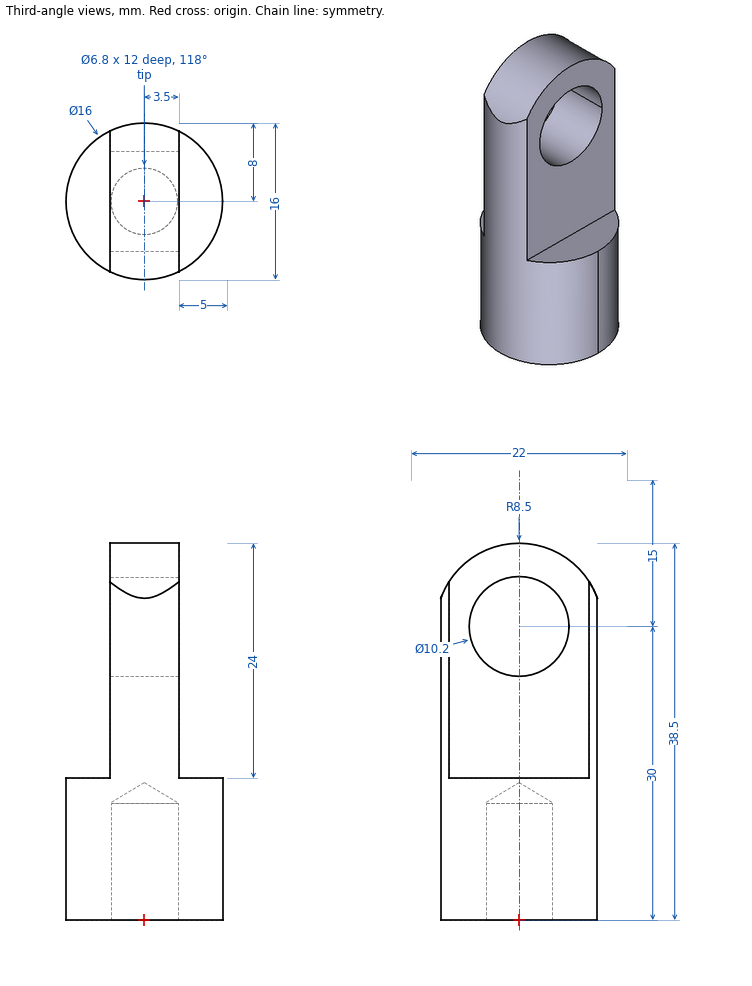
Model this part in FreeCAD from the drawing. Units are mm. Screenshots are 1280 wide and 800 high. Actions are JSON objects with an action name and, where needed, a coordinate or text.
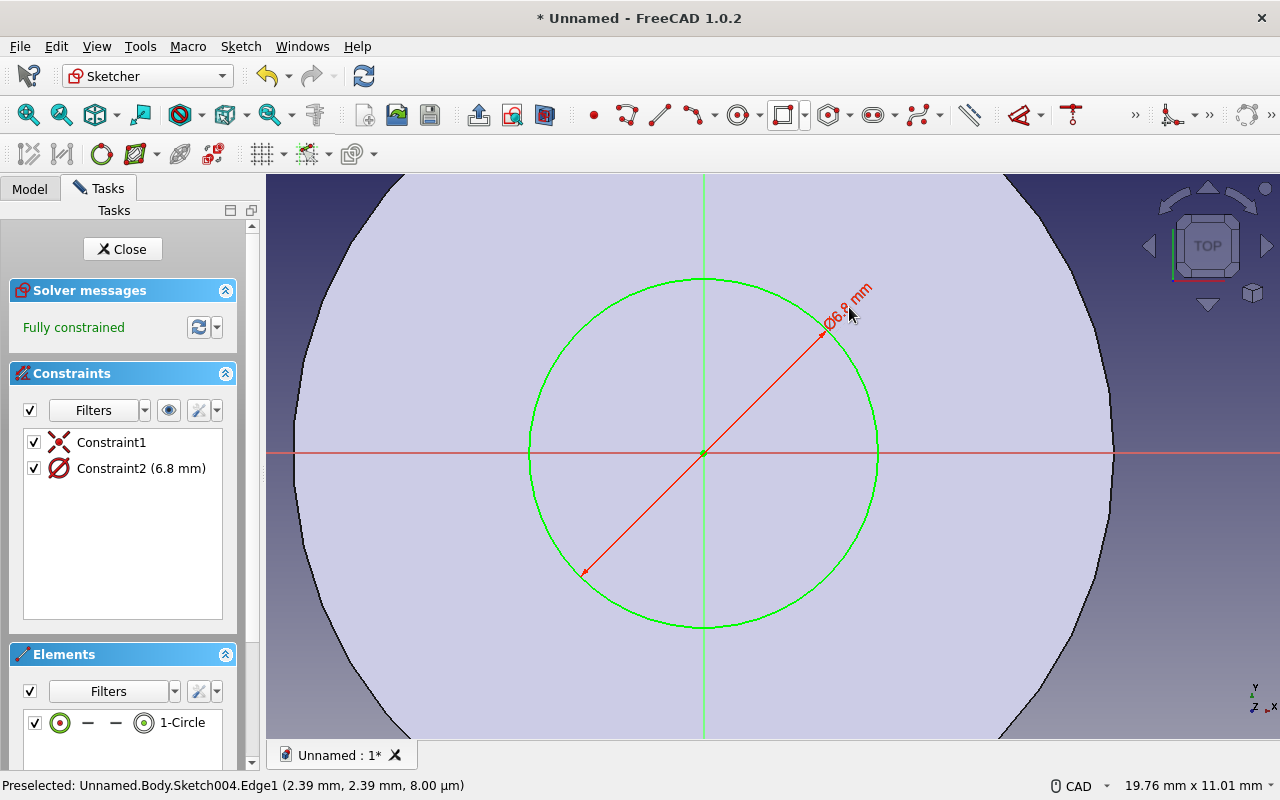
{"action": "left_click", "coordinate": [123, 249]}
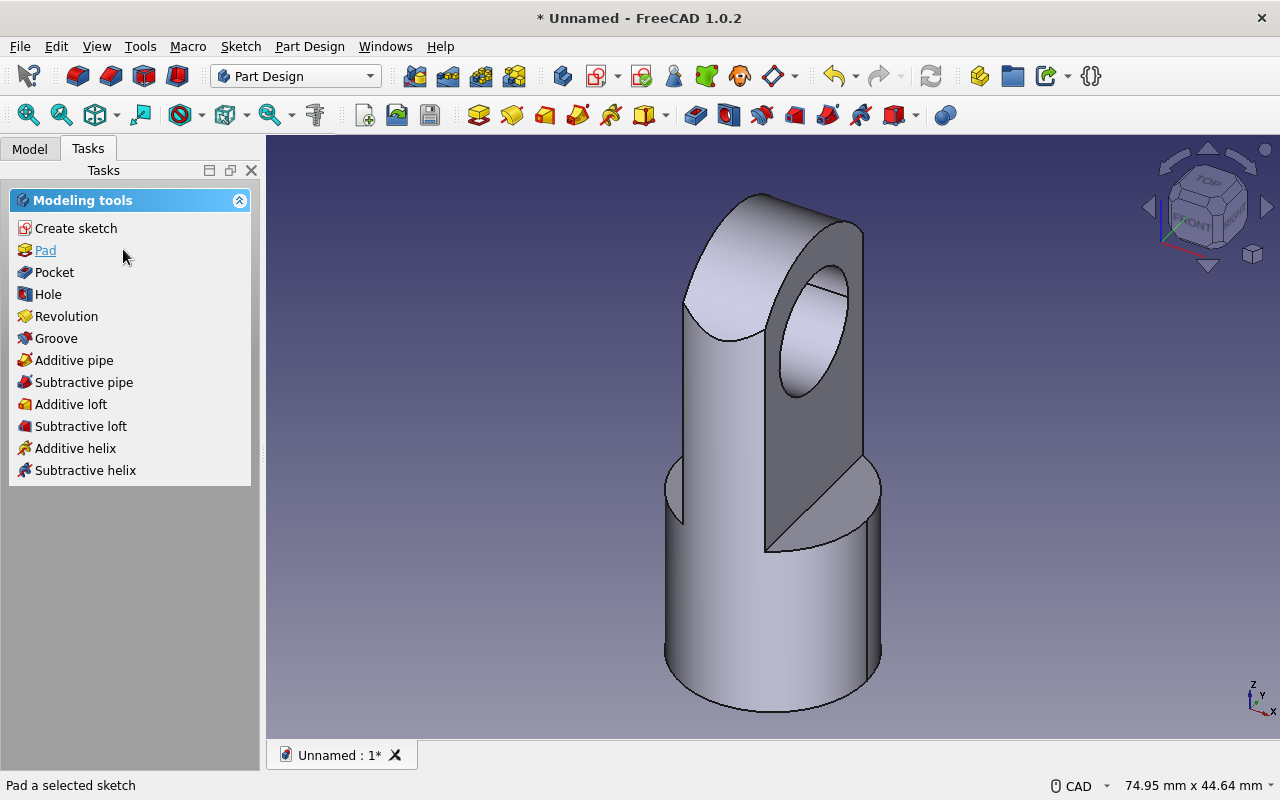
{"action": "left_click", "coordinate": [729, 116]}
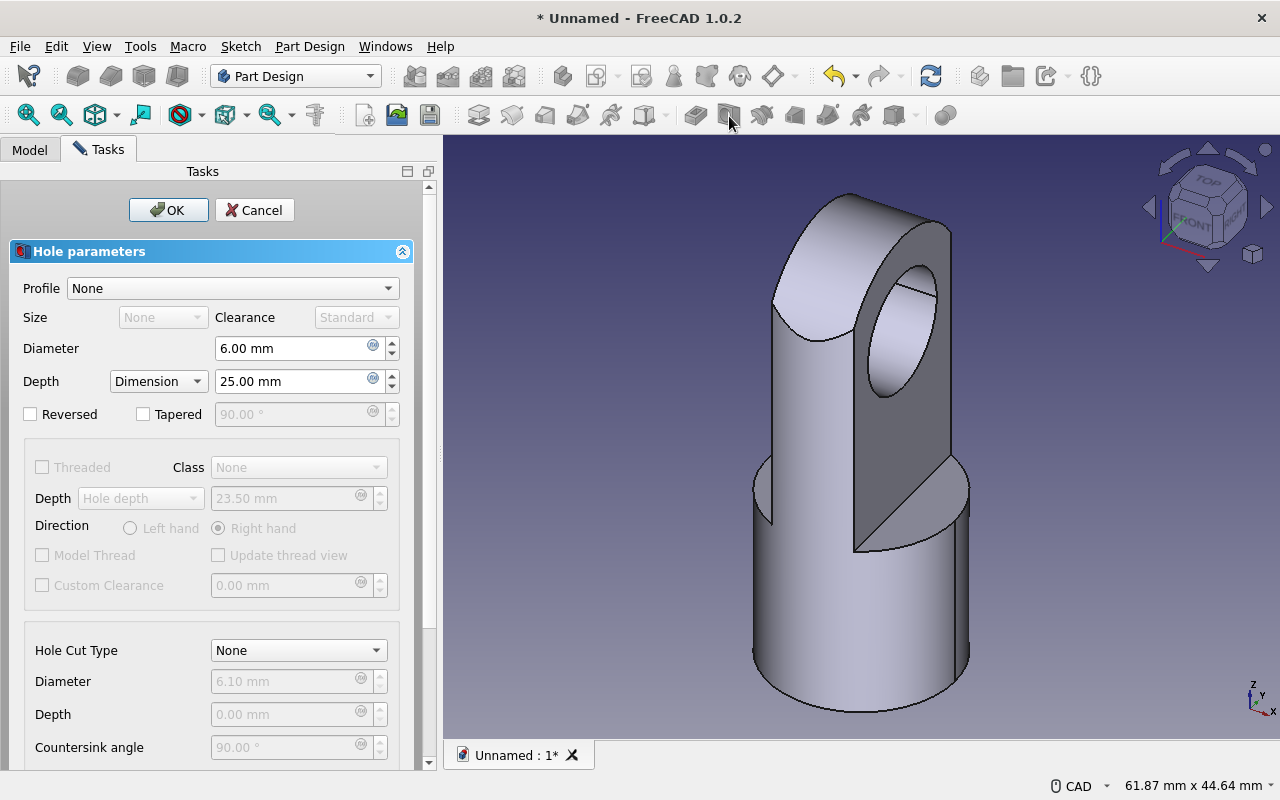
{"action": "triple_click", "coordinate": [300, 348]}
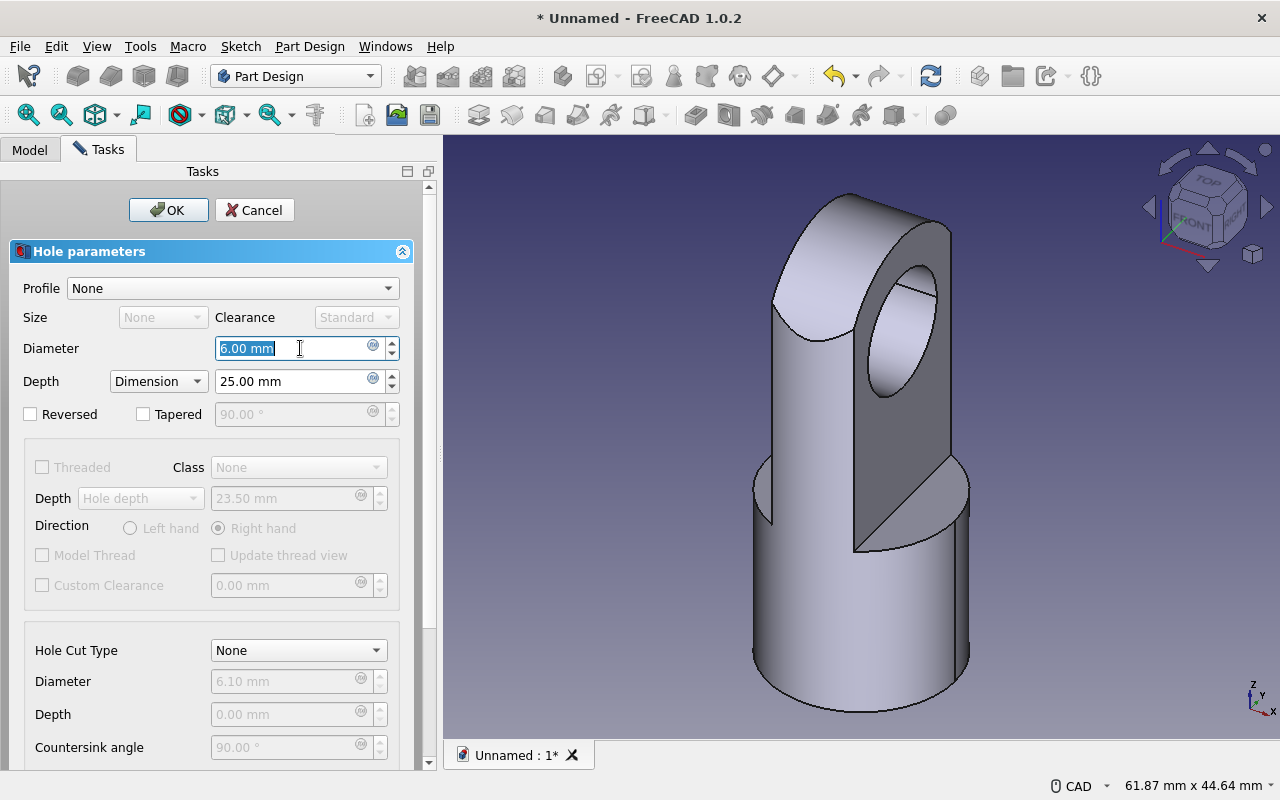
{"action": "type", "text": "6.8"}
{"action": "key", "text": "Tab"}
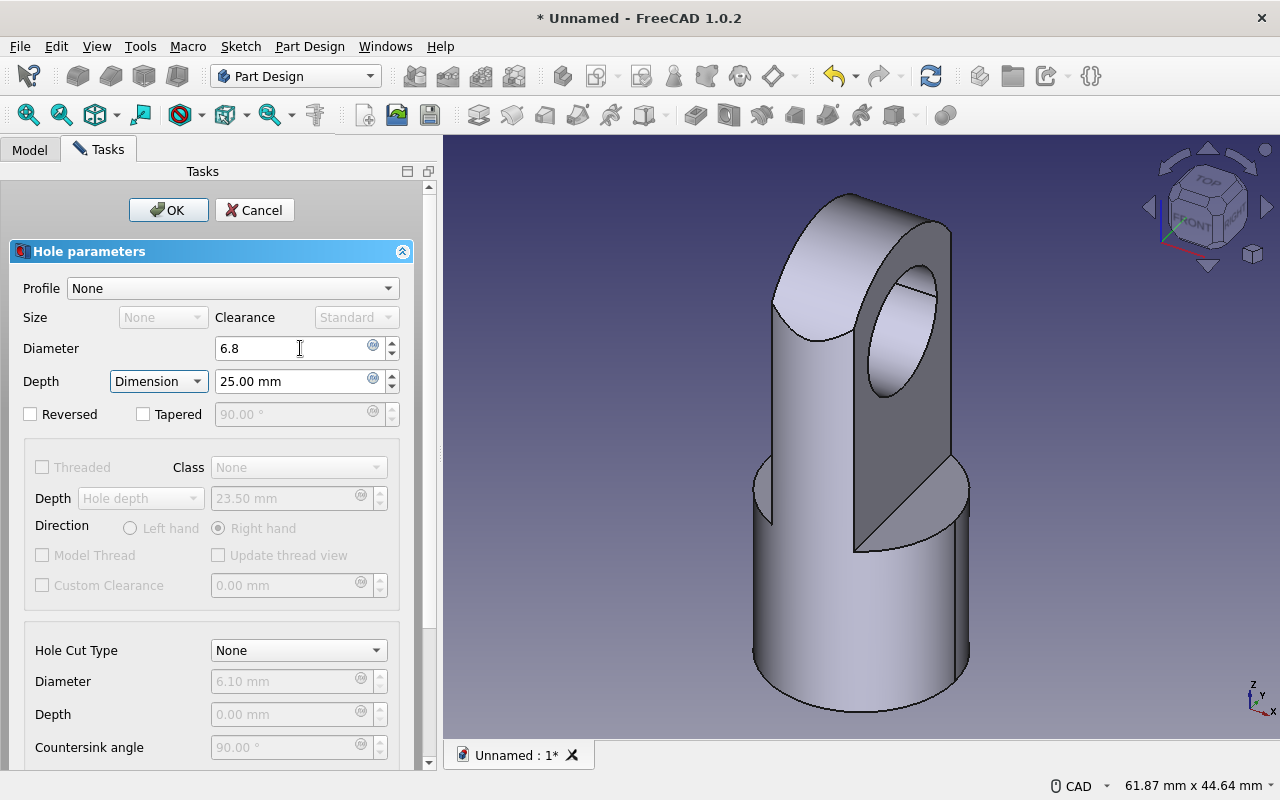
{"action": "triple_click", "coordinate": [300, 382]}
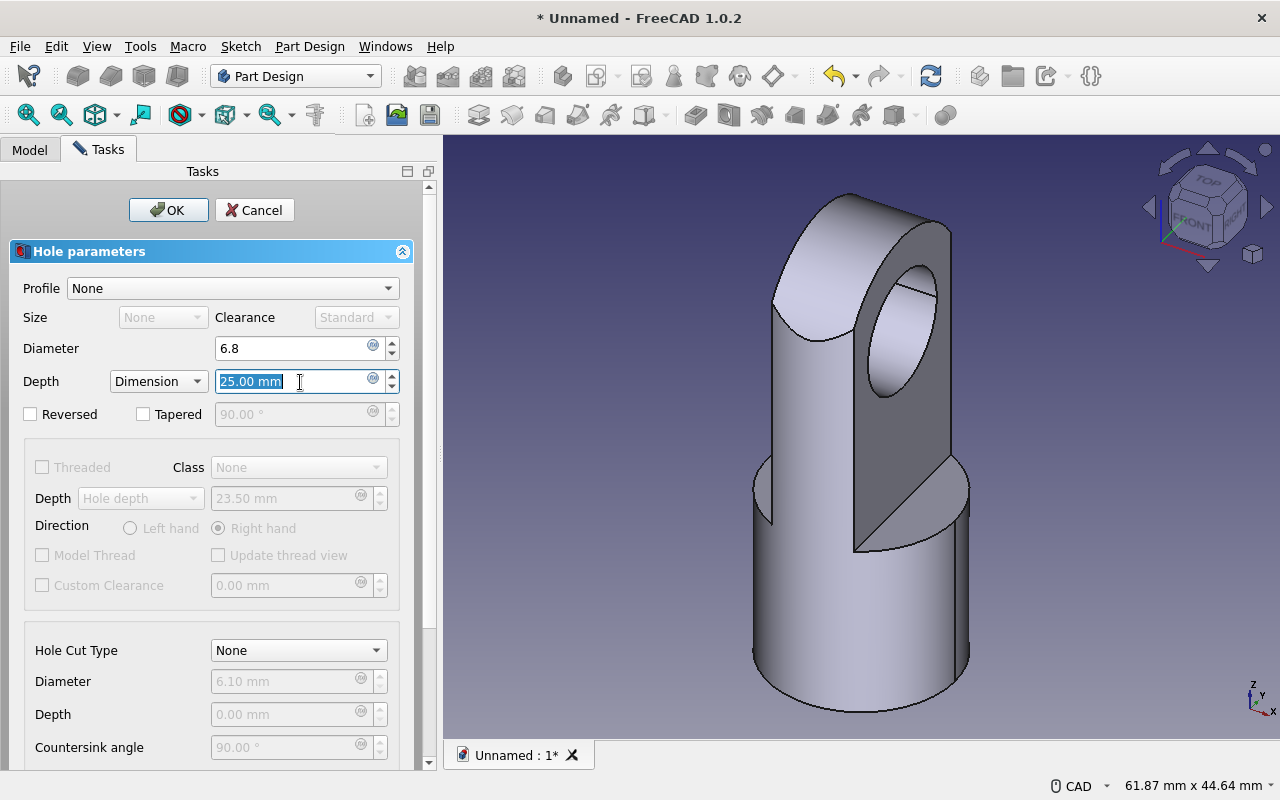
{"action": "type", "text": "12"}
{"action": "key", "text": "Tab"}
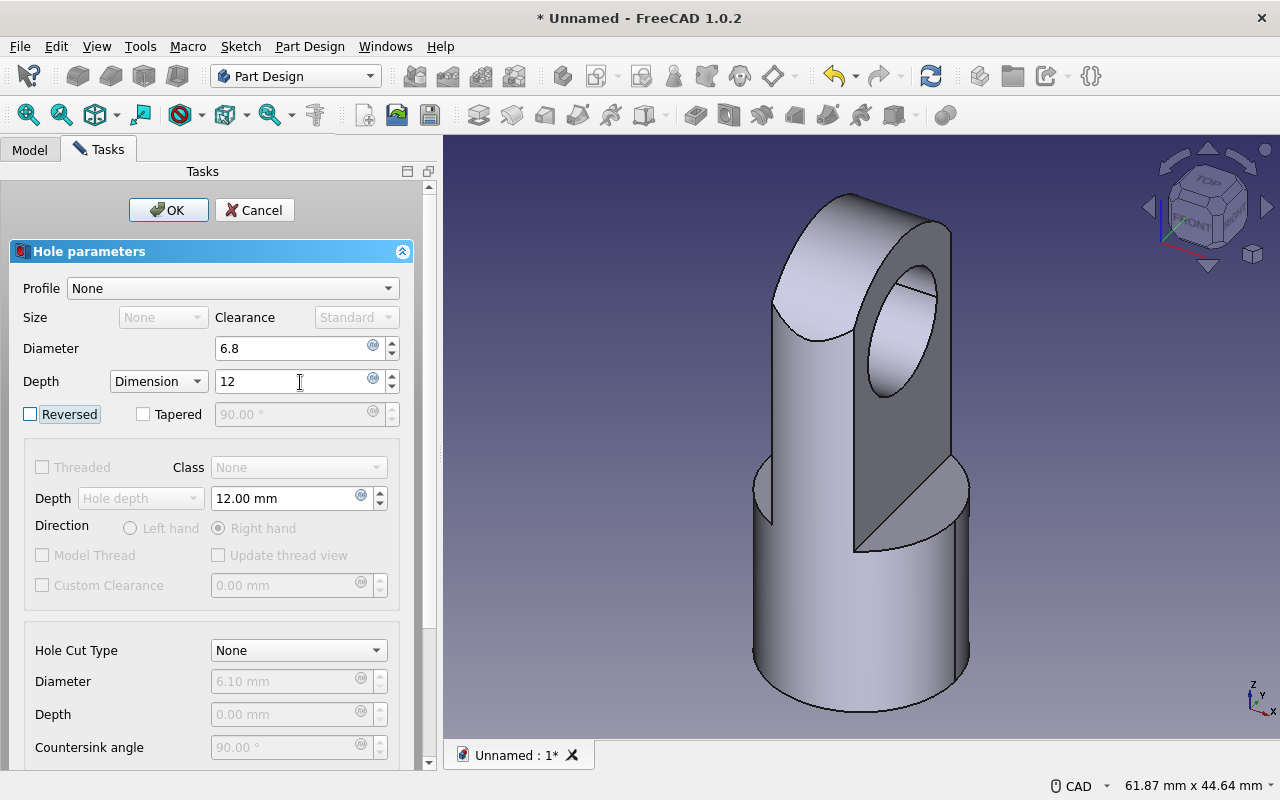
{"action": "left_click", "coordinate": [31, 414]}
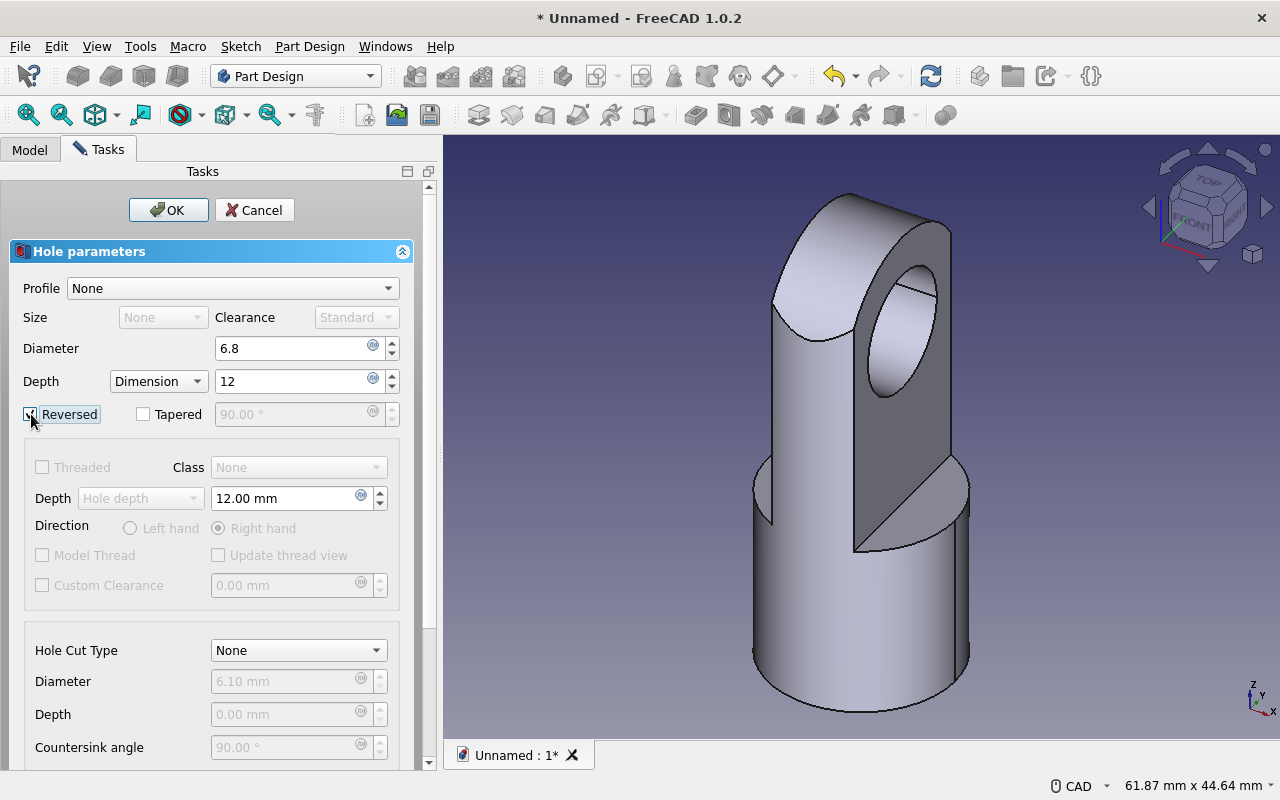
{"action": "left_click", "coordinate": [169, 210]}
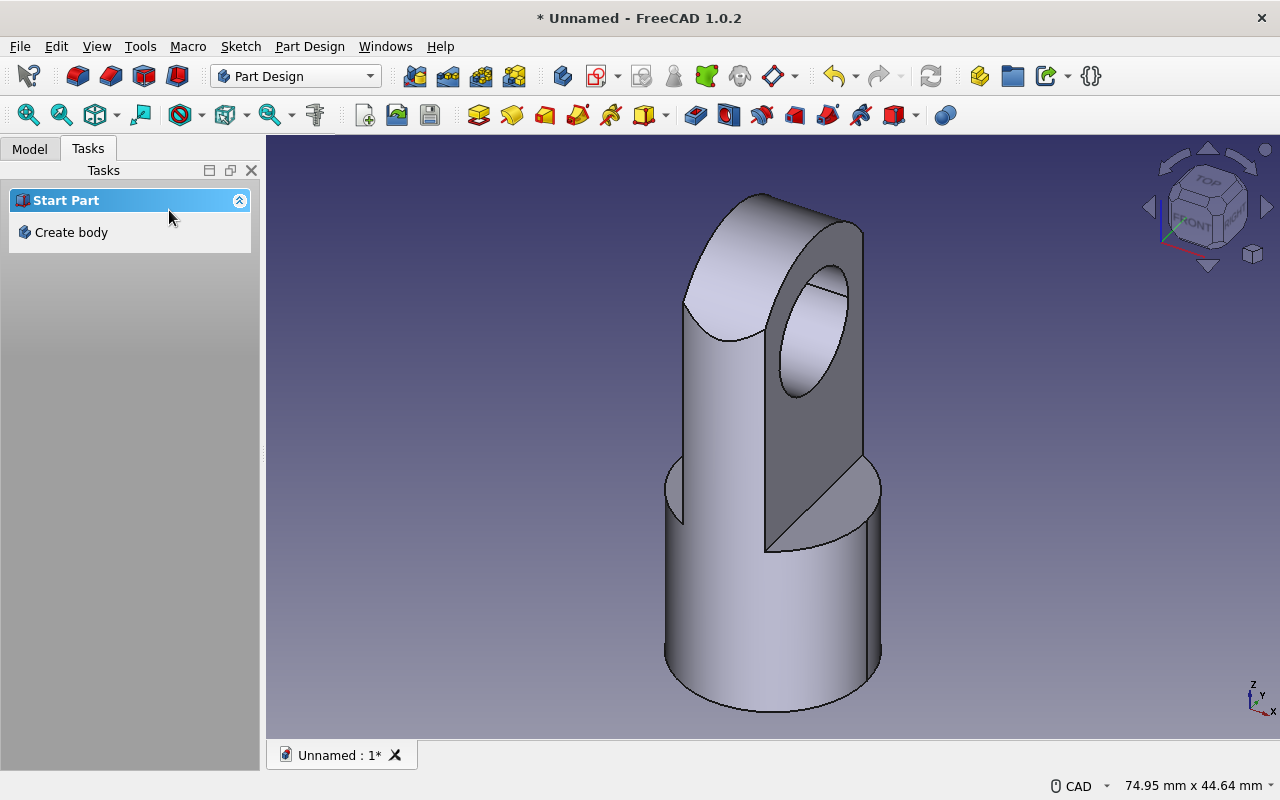
{"action": "key", "text": "0"}